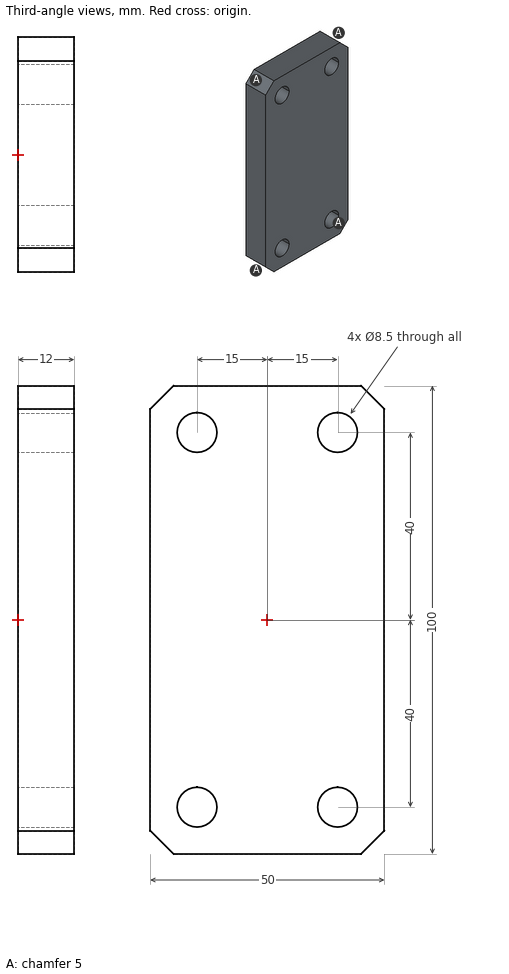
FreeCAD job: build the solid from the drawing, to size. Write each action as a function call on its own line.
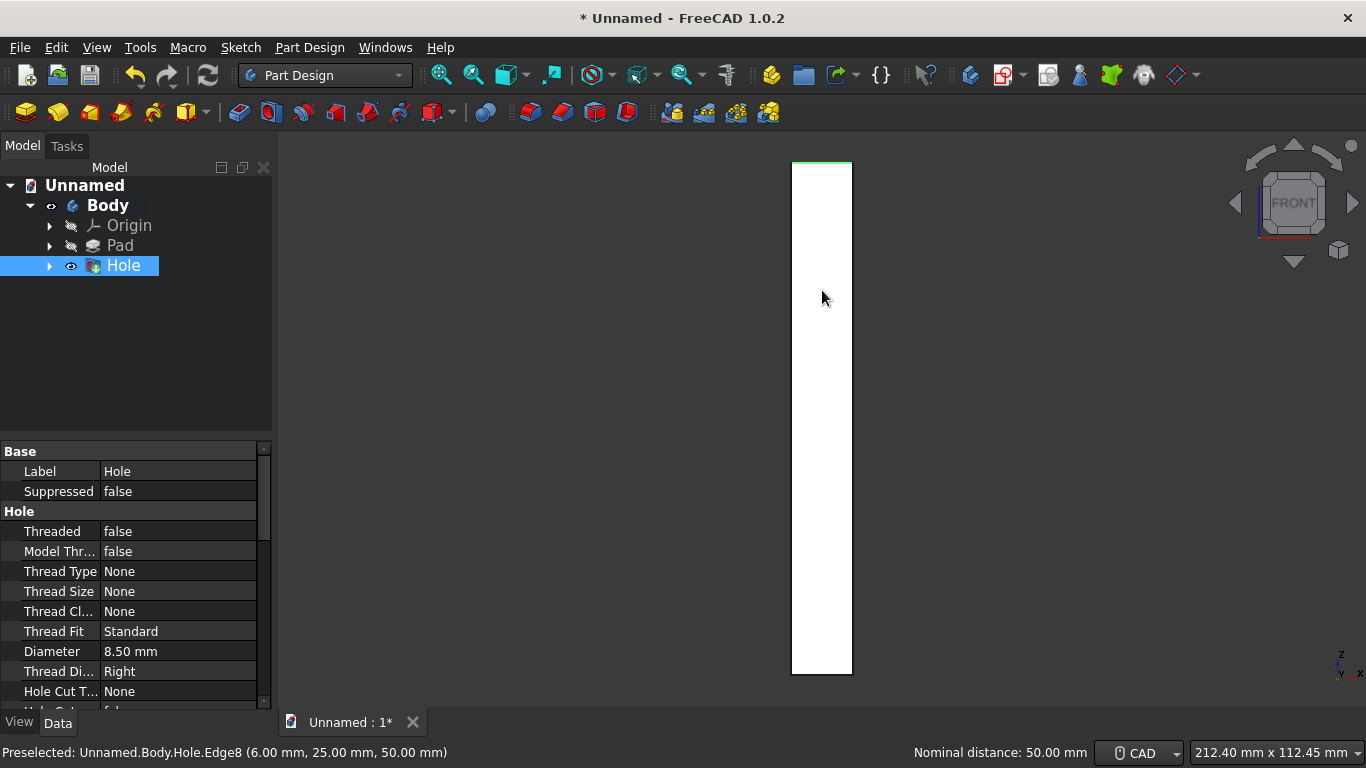
click(822, 674, ctrl)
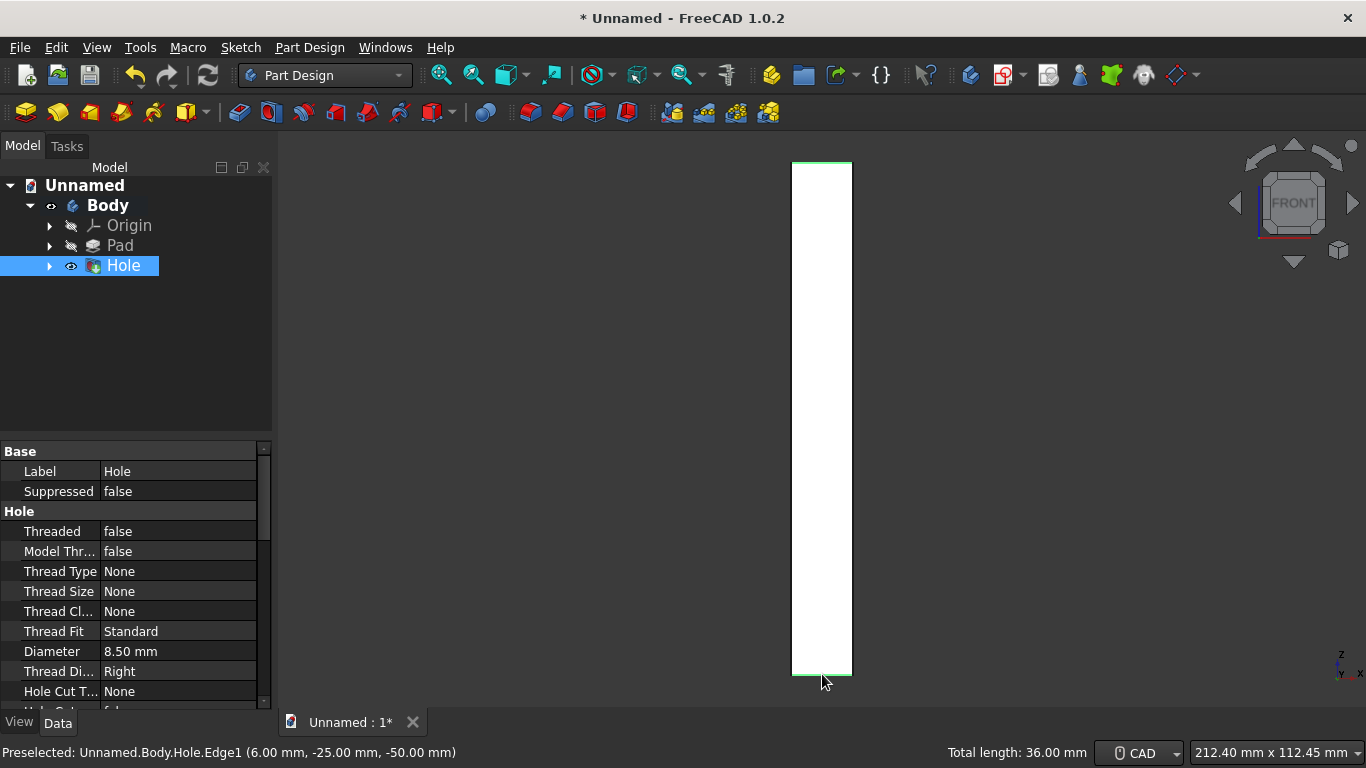
key(3)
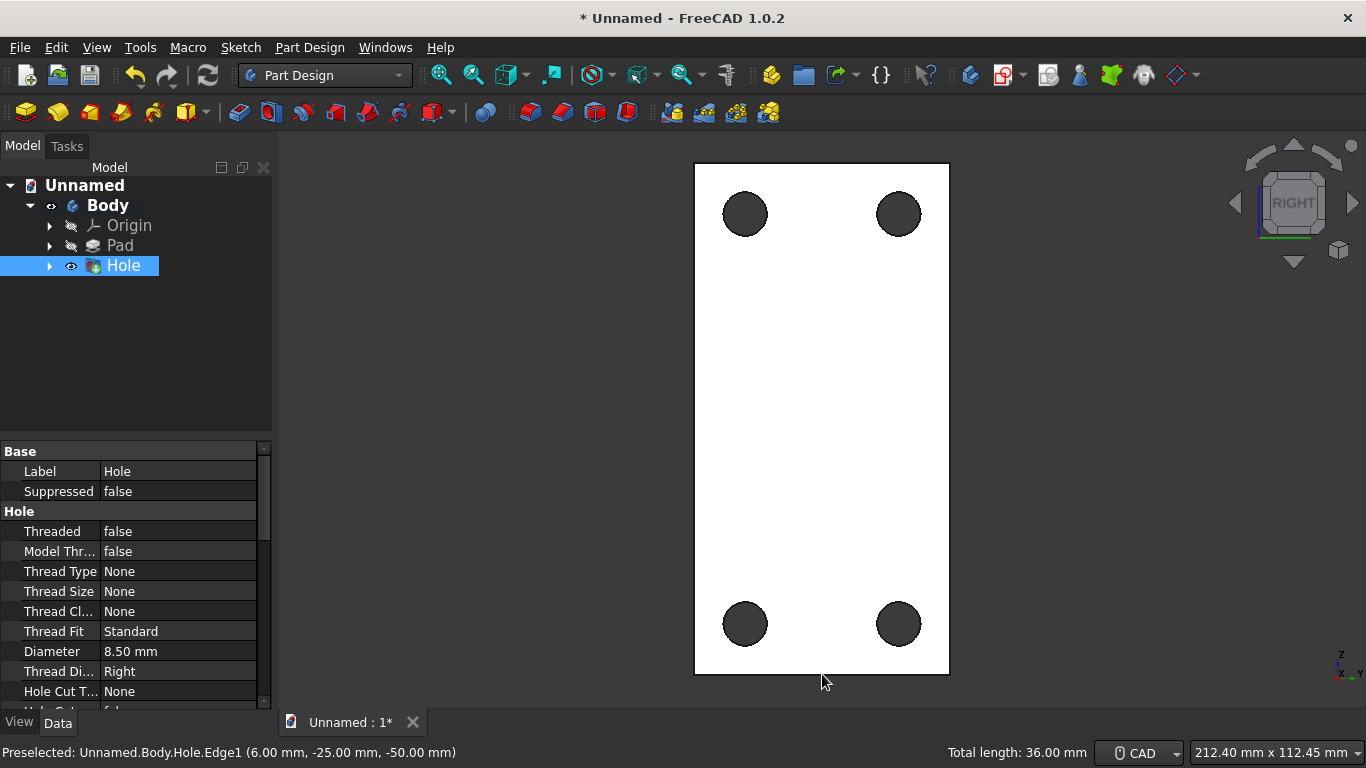
key(5)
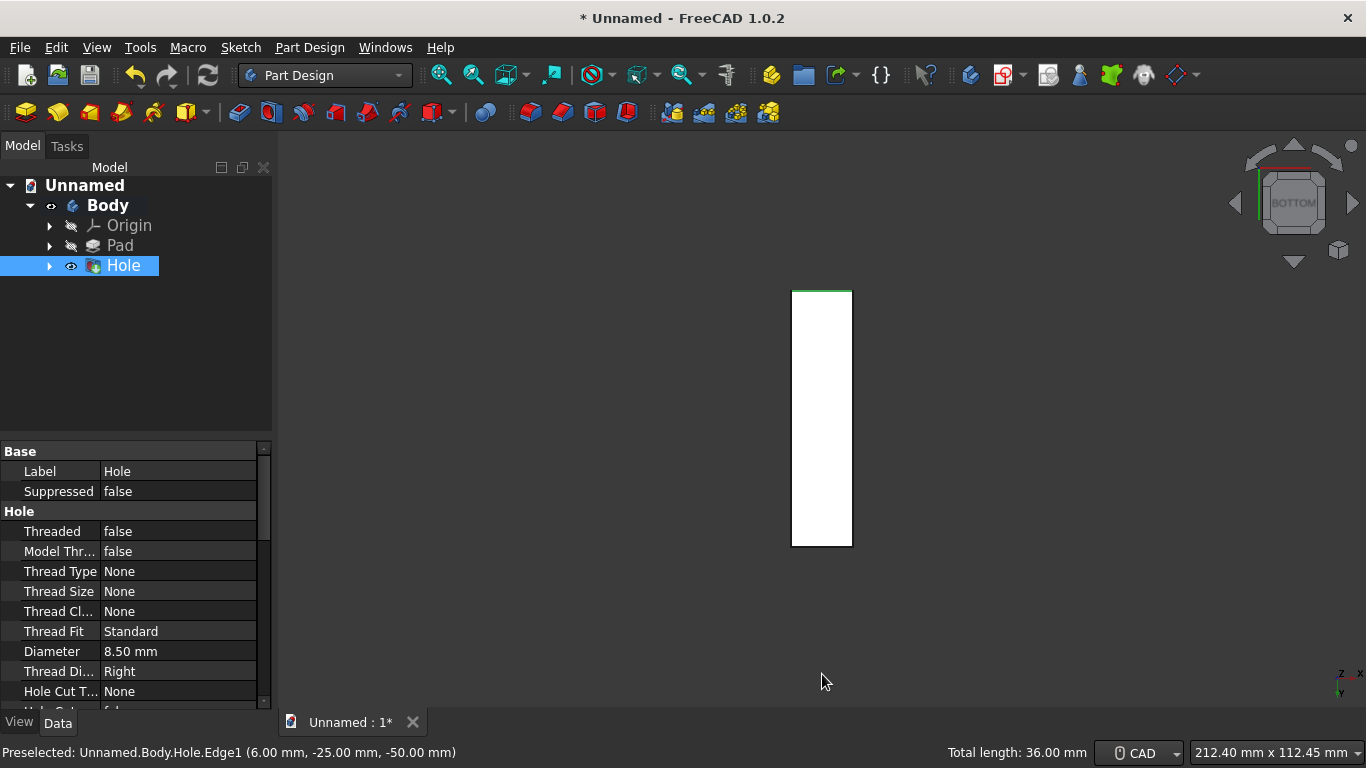
click(442, 76)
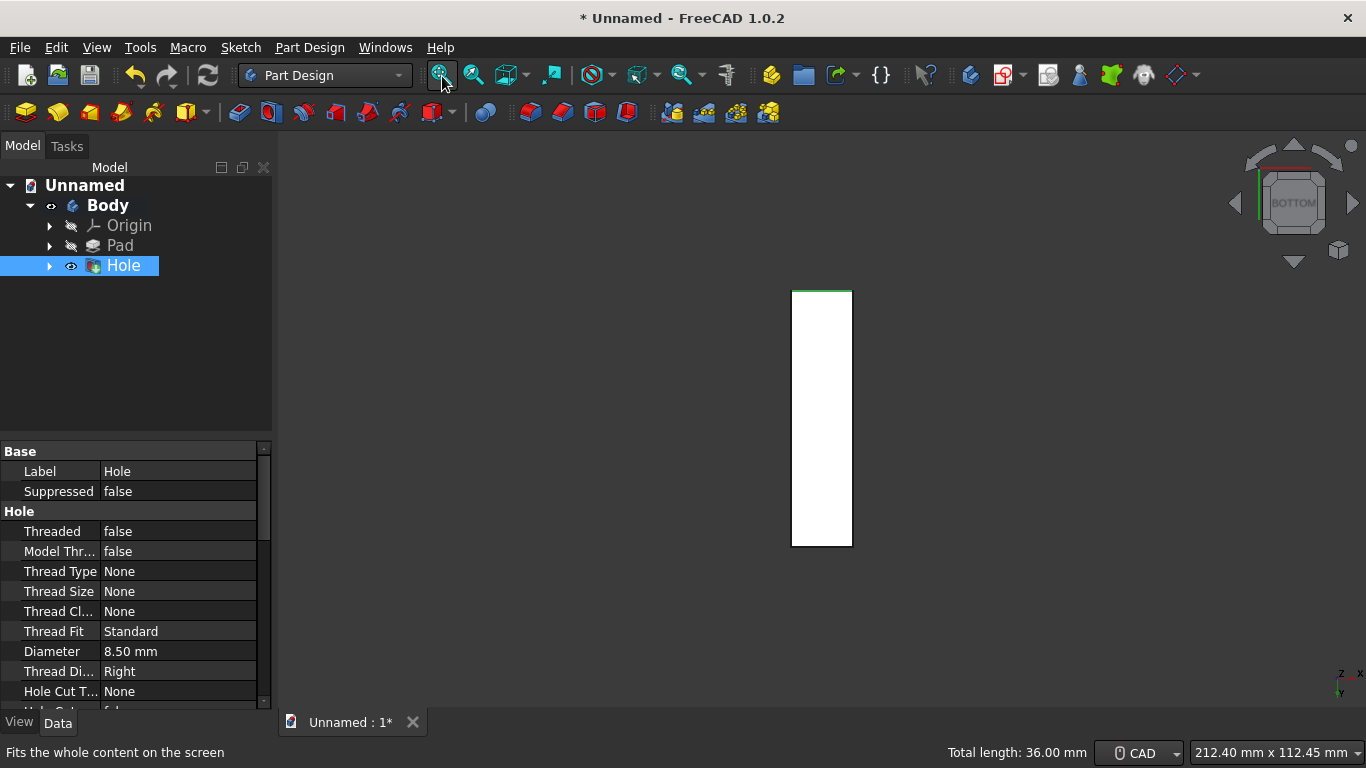
click(822, 546, ctrl)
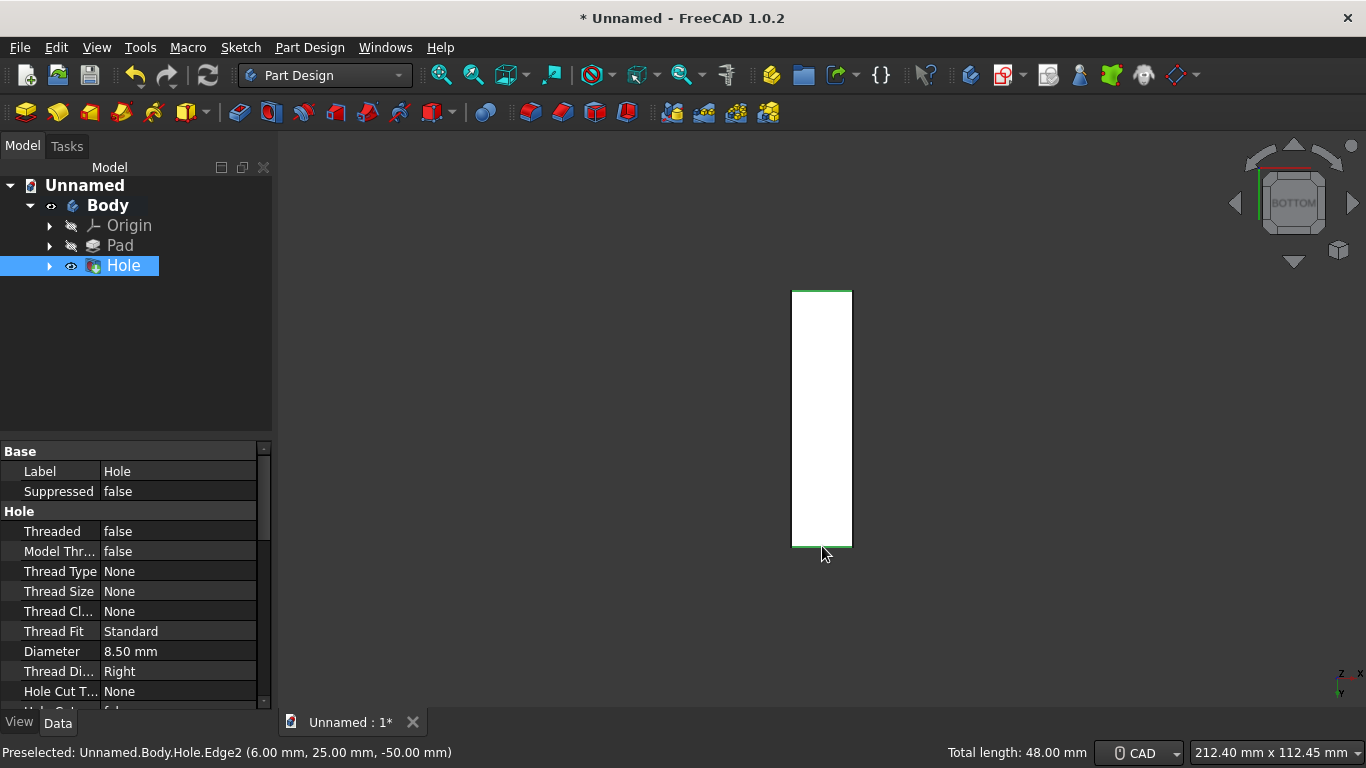
click(564, 112)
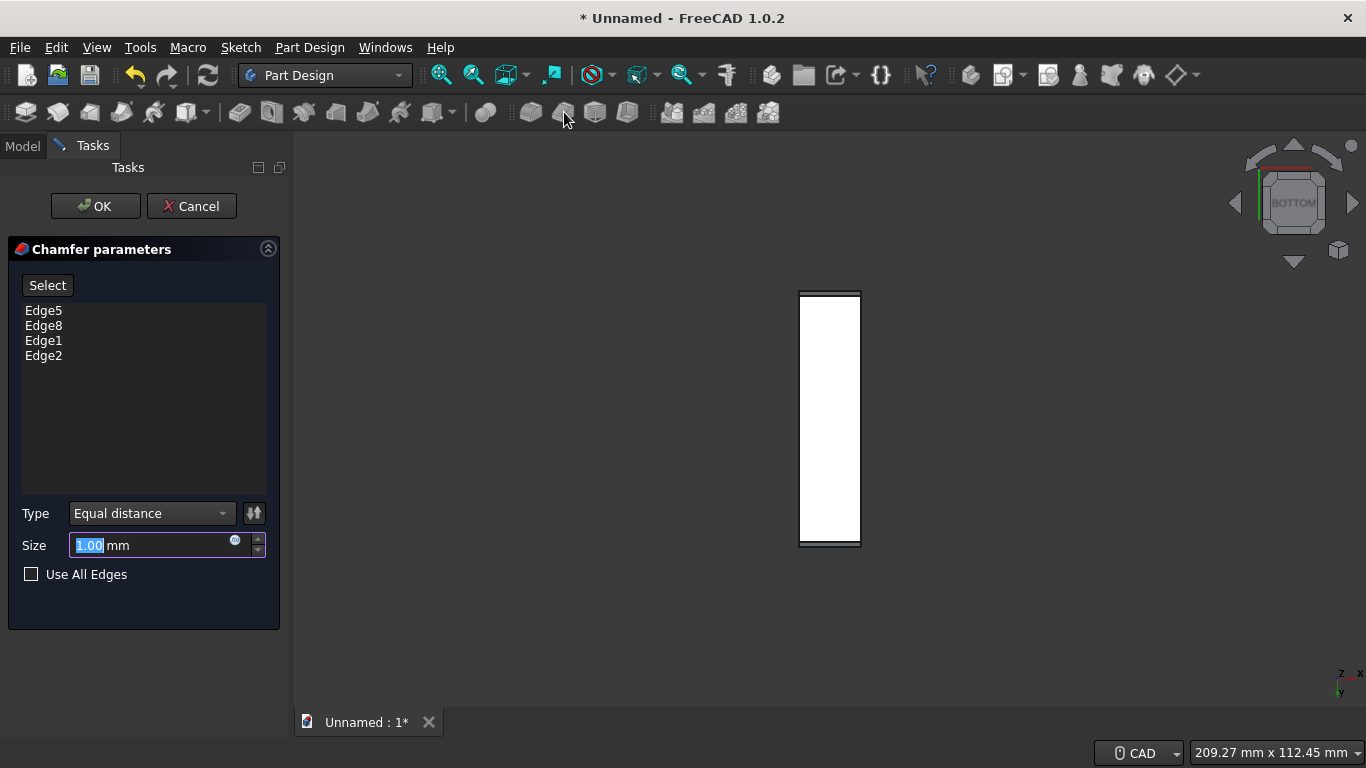
text(5)
key(Tab)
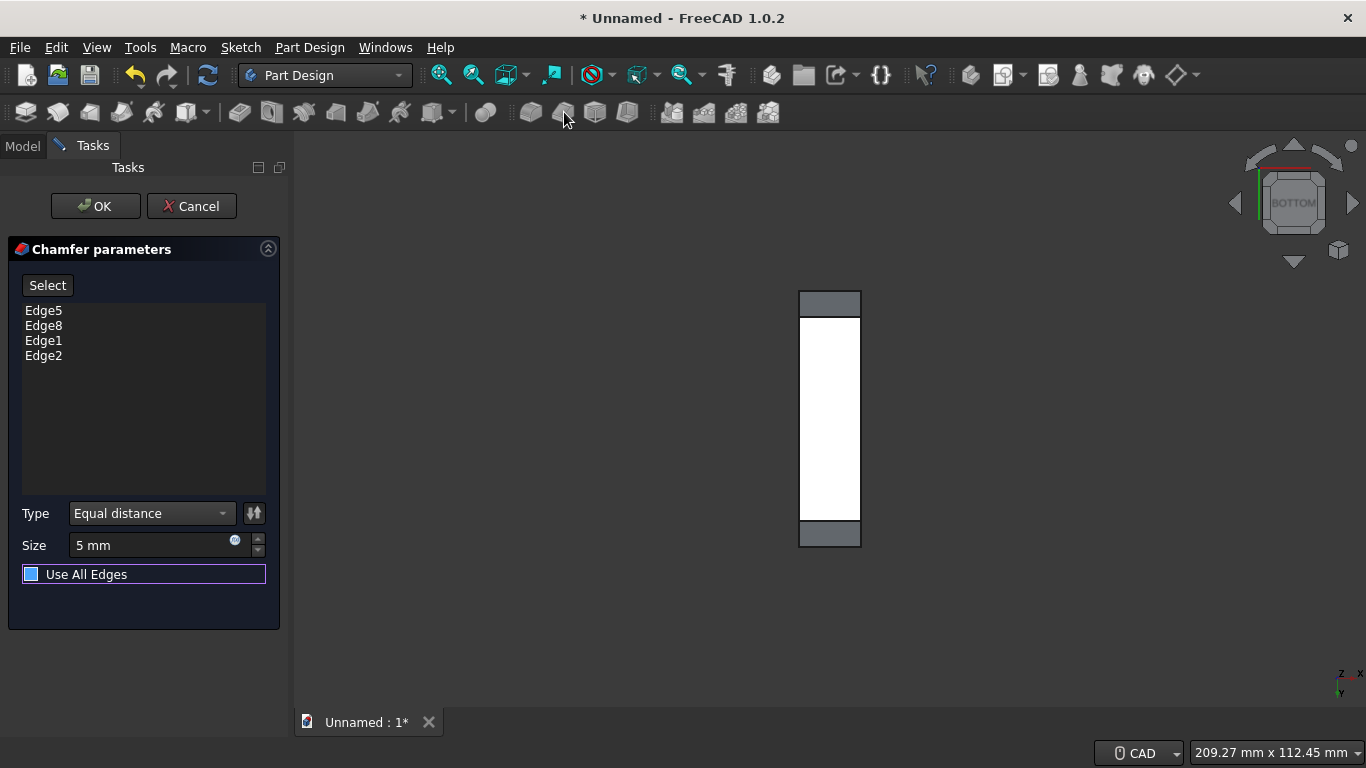
click(96, 206)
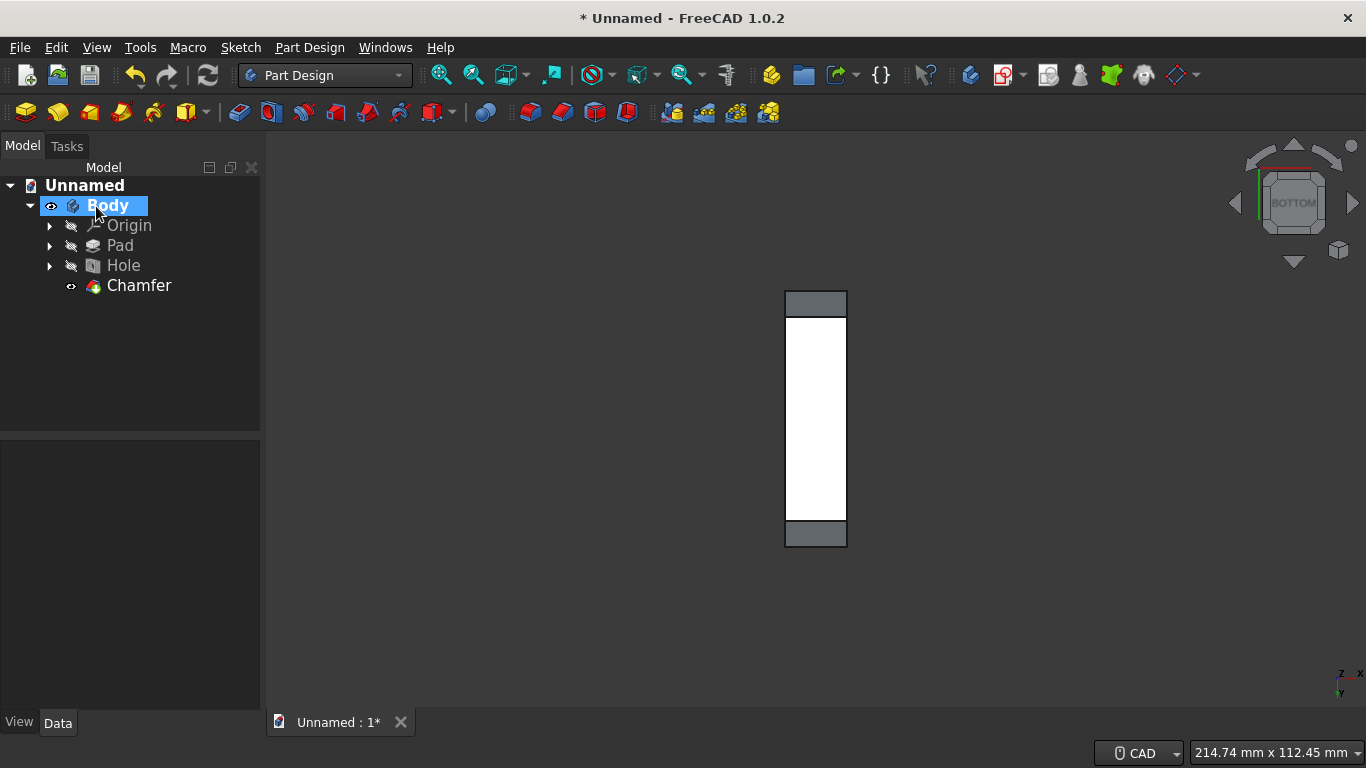
key(0)